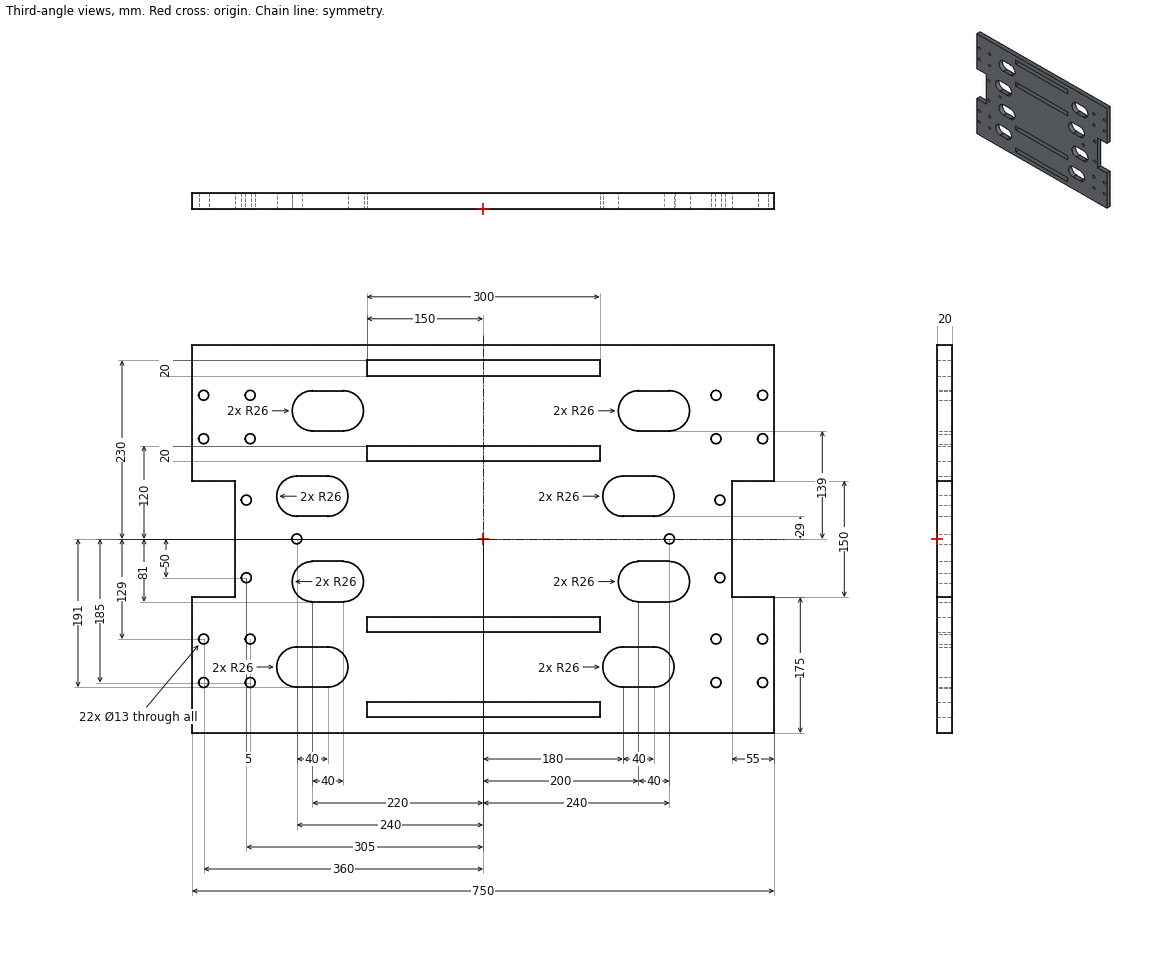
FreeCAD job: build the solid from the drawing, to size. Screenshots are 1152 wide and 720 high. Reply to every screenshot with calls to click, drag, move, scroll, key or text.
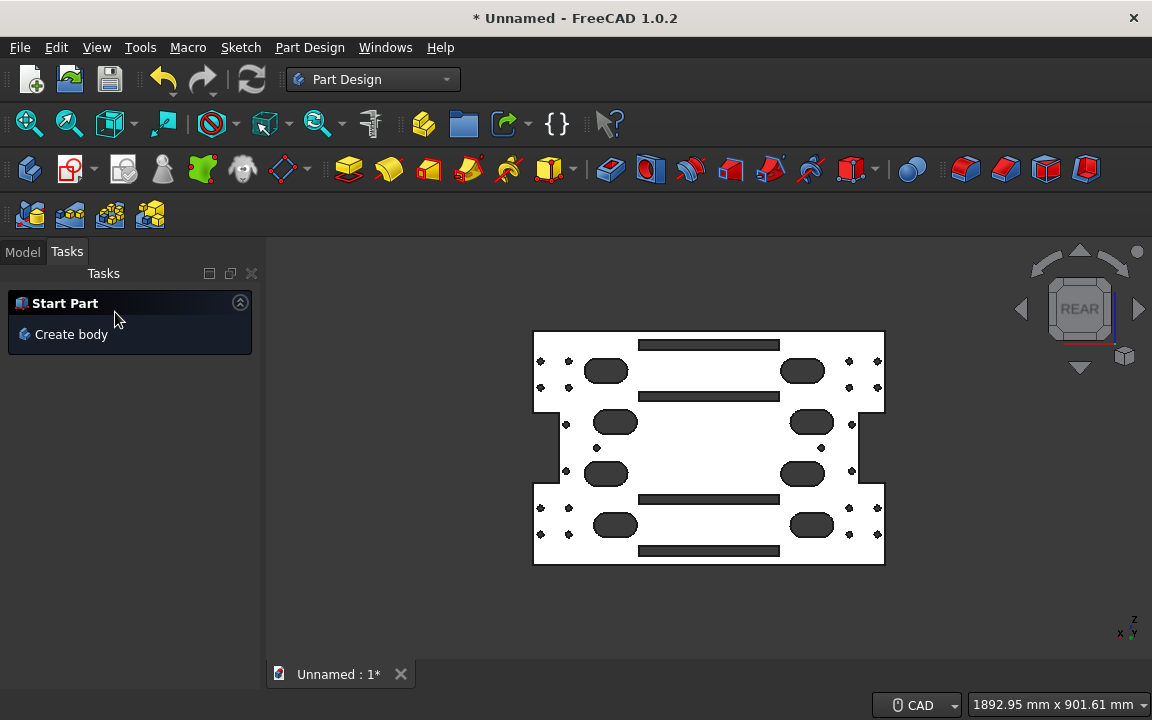
key(0)